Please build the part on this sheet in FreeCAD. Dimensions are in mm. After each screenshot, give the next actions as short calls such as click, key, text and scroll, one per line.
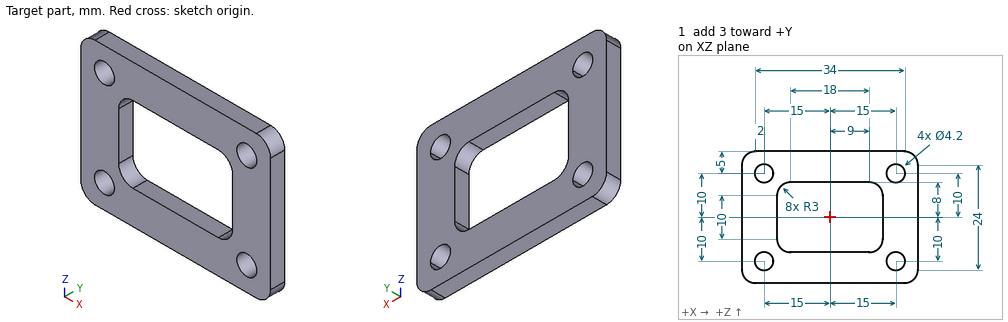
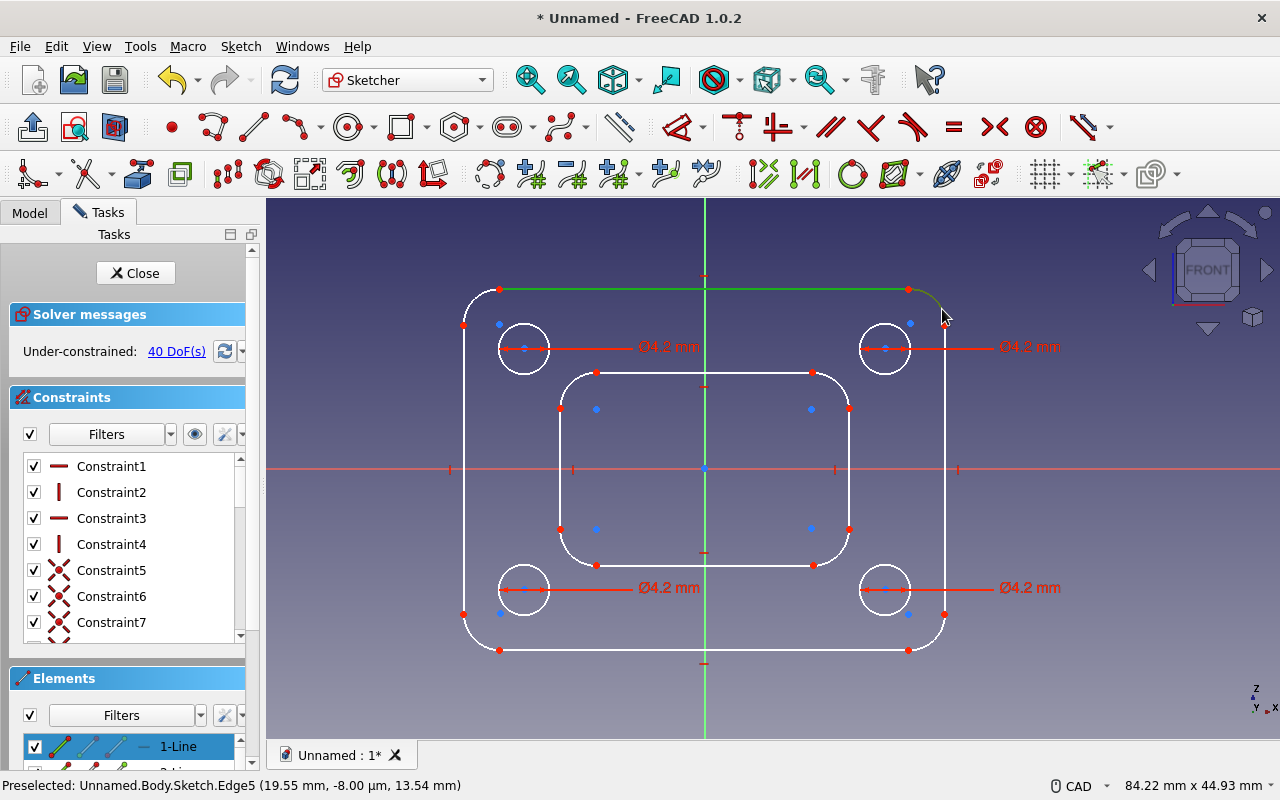
key(t)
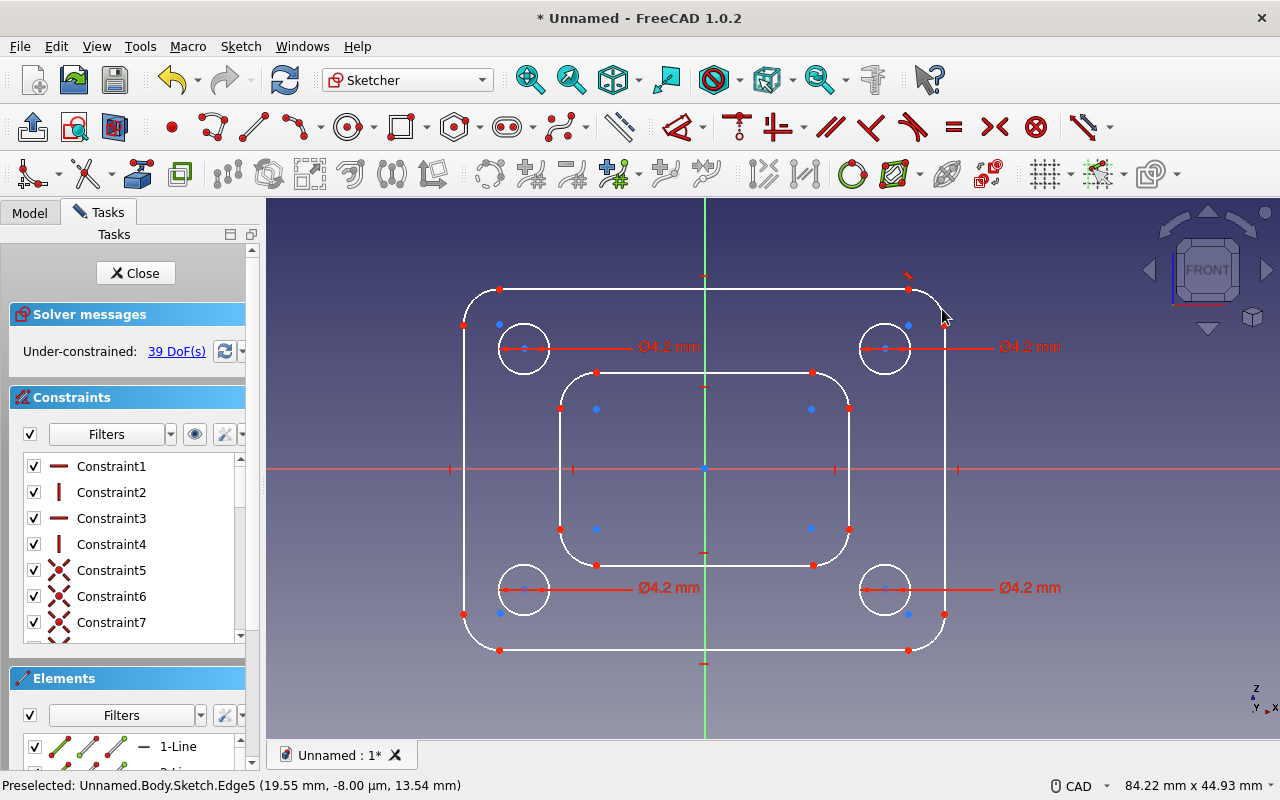
click(623, 289)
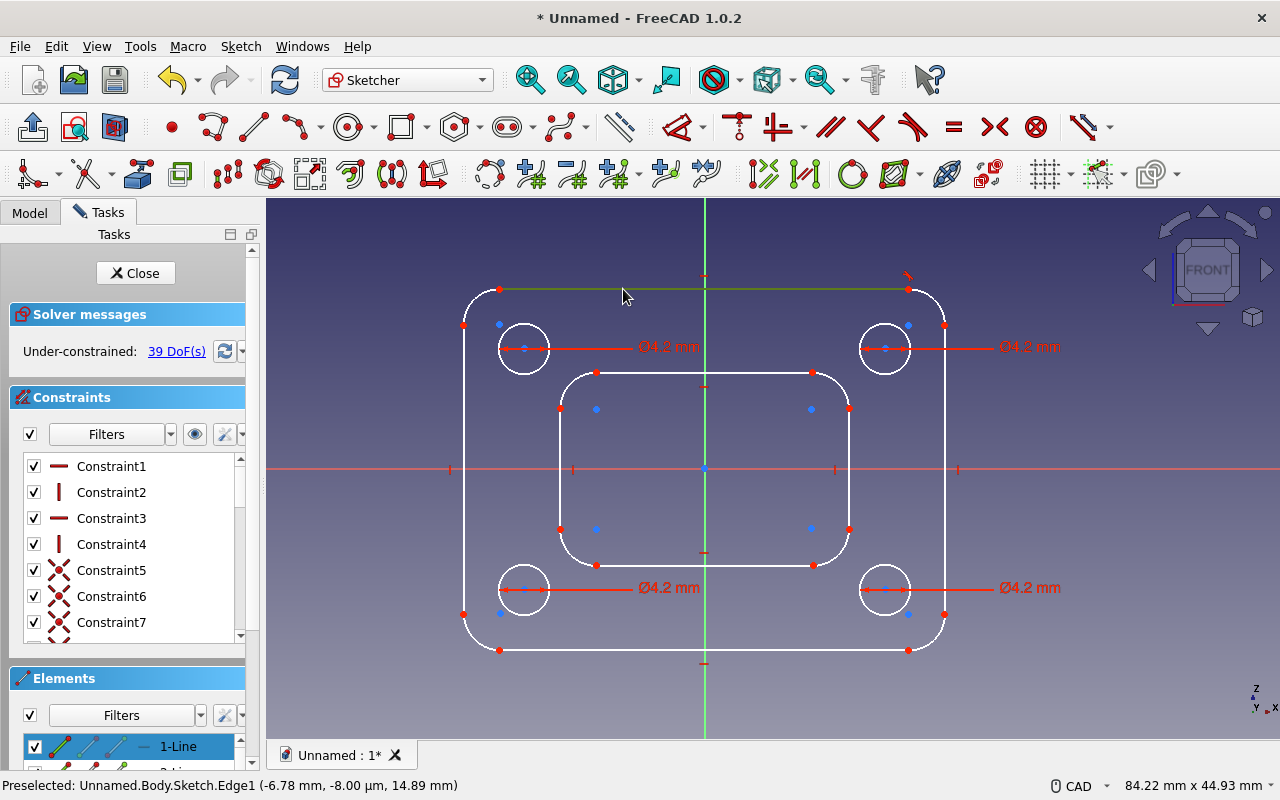
click(483, 293)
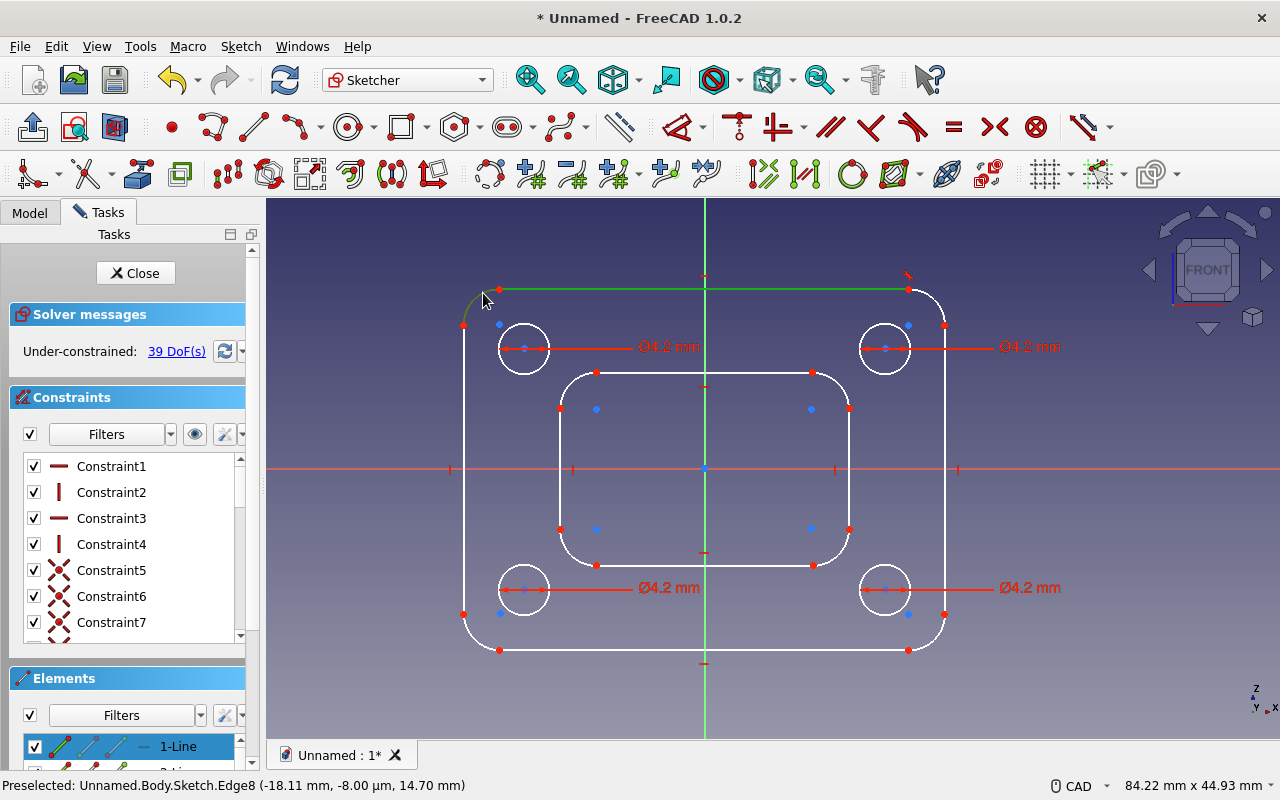
click(913, 128)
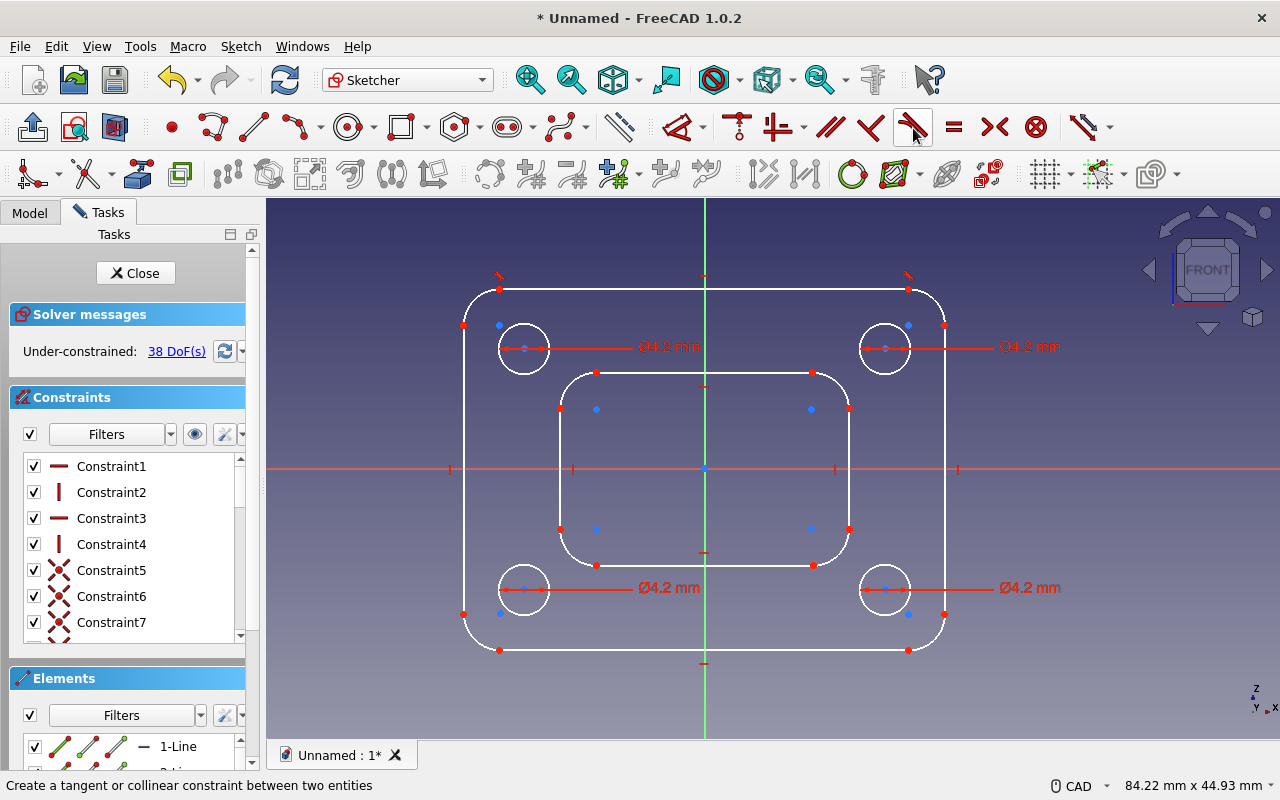
click(945, 412)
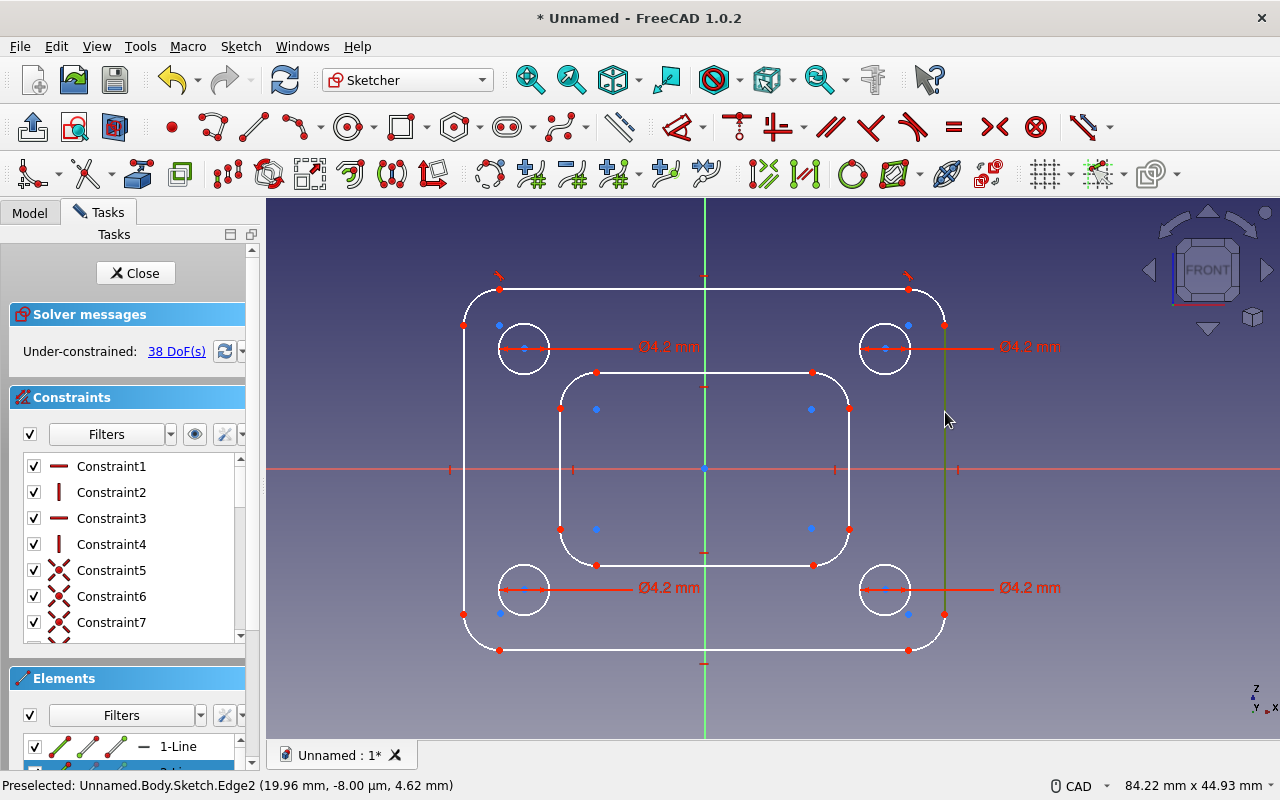
click(941, 309)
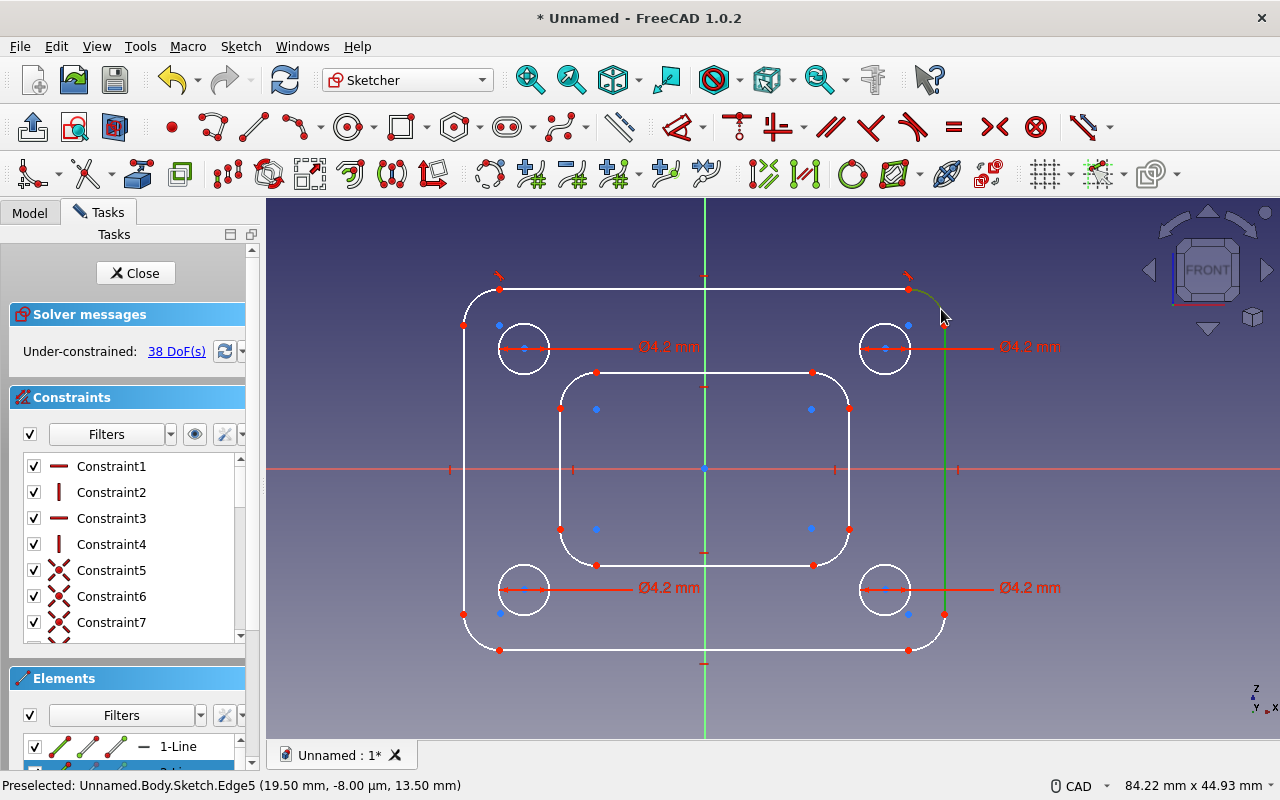
key(t)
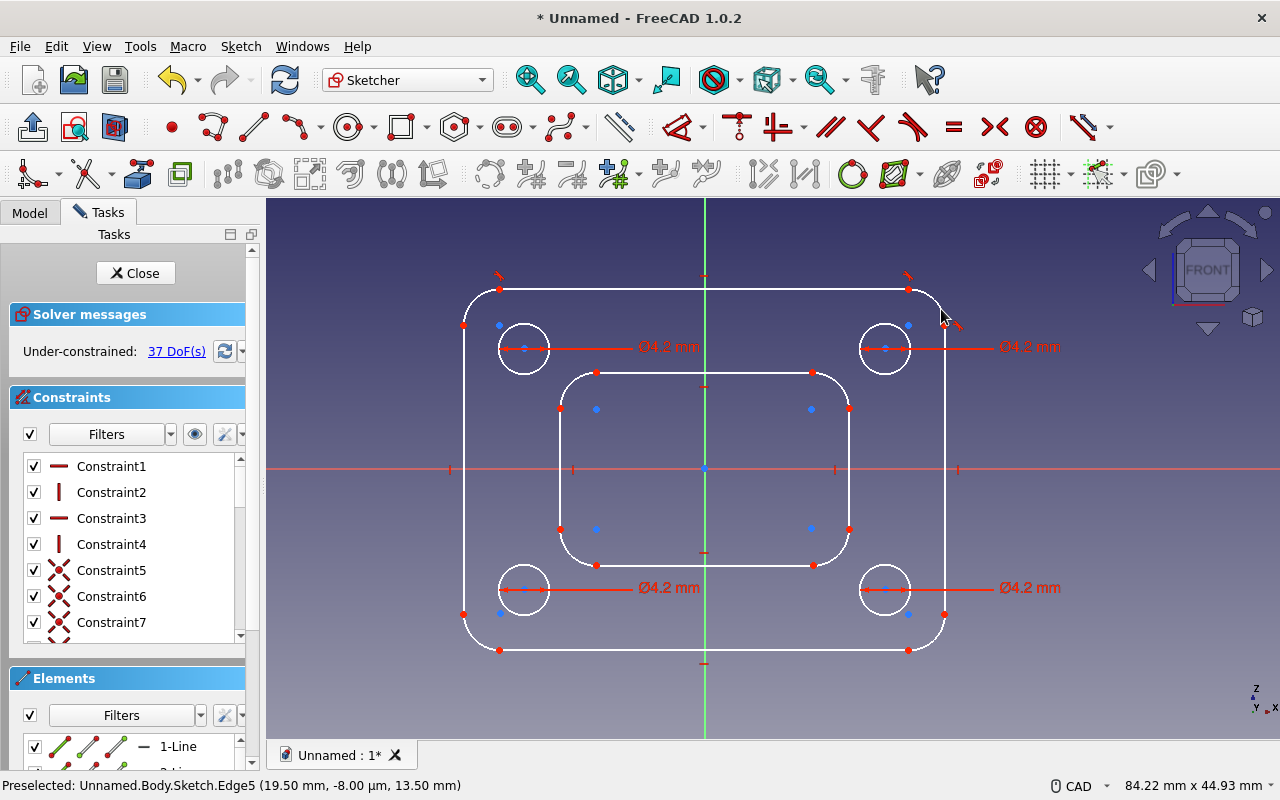
click(945, 412)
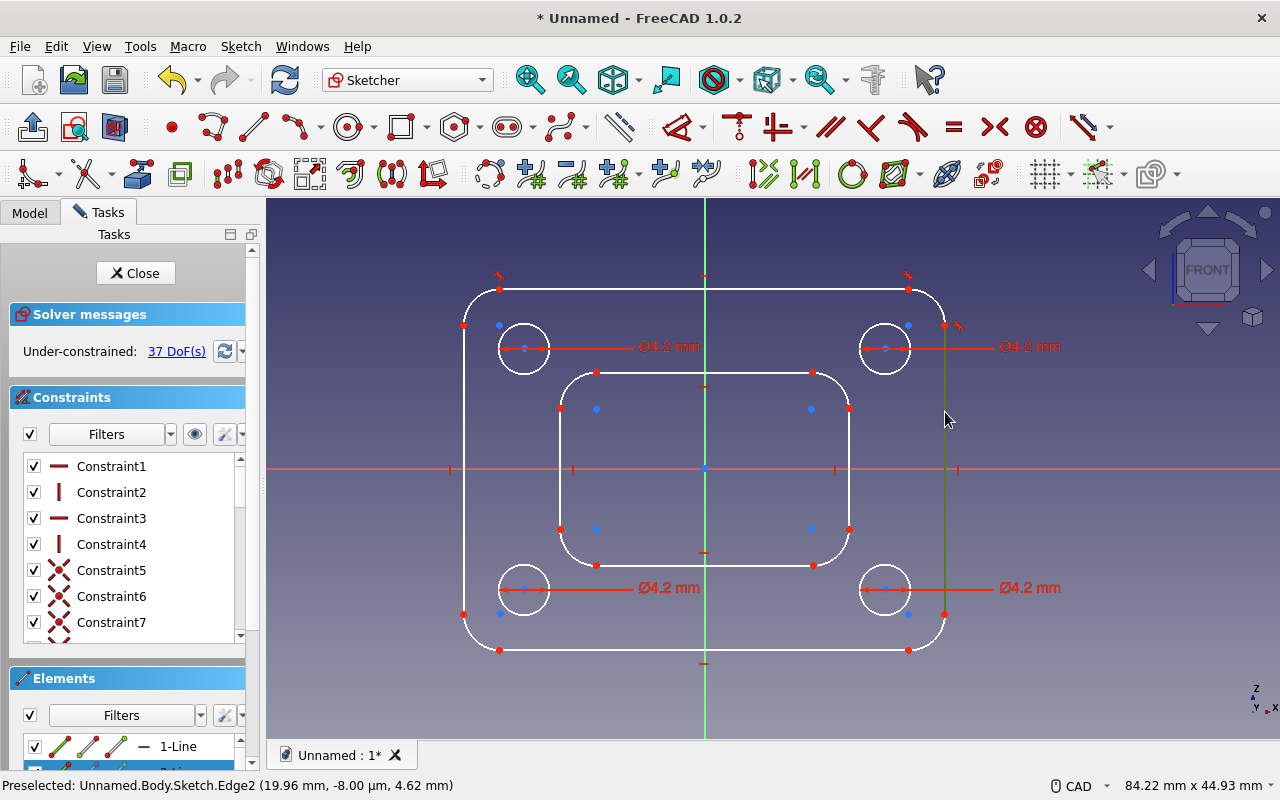
click(925, 646)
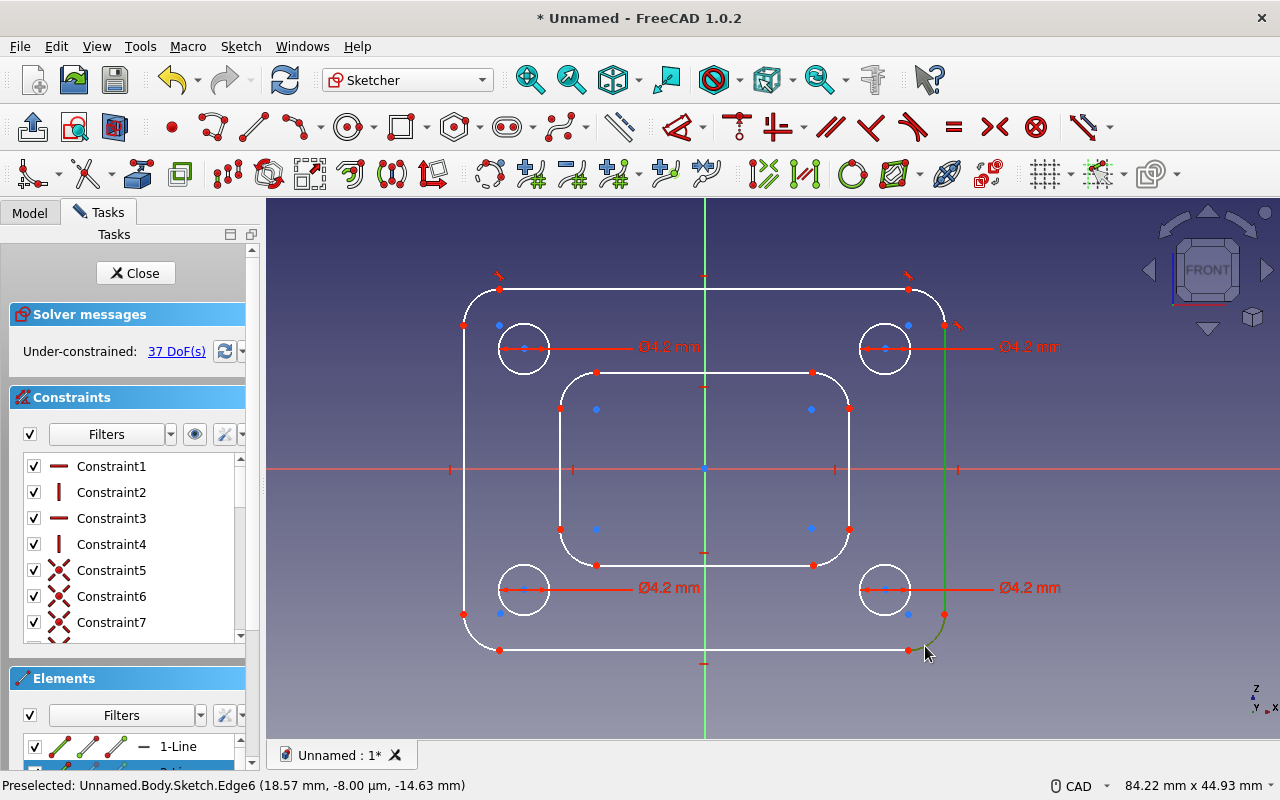
key(t)